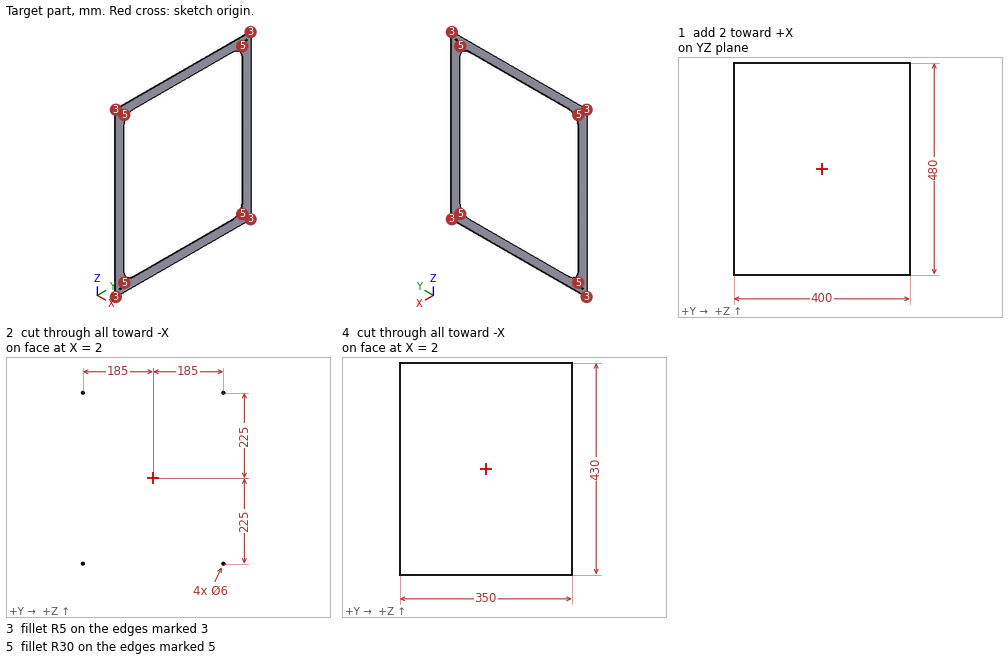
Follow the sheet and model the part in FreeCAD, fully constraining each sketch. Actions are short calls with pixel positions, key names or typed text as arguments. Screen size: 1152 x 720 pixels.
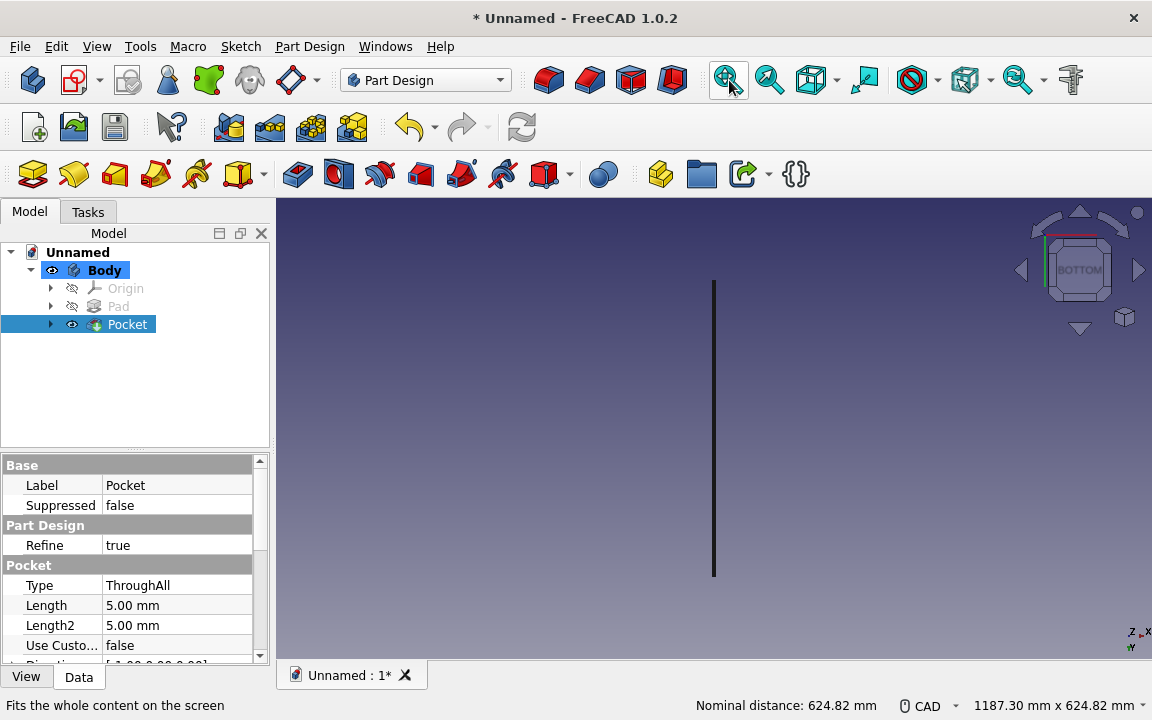
scroll(714, 575, up, 15)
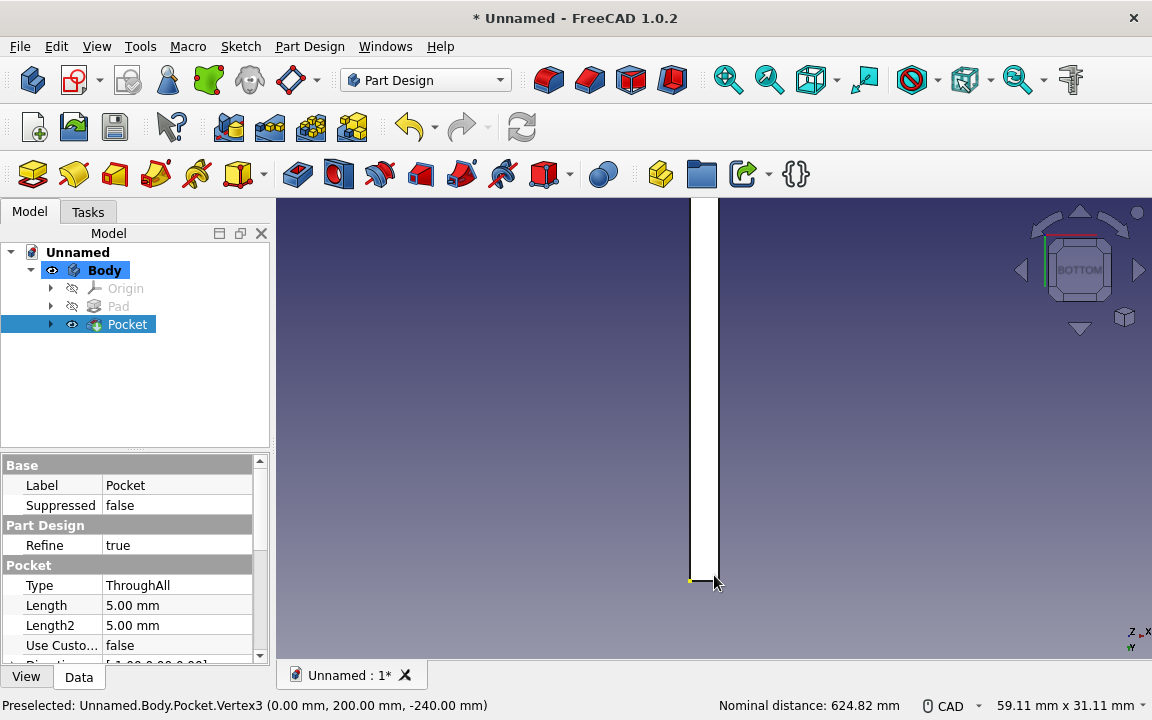
click(704, 580, ctrl)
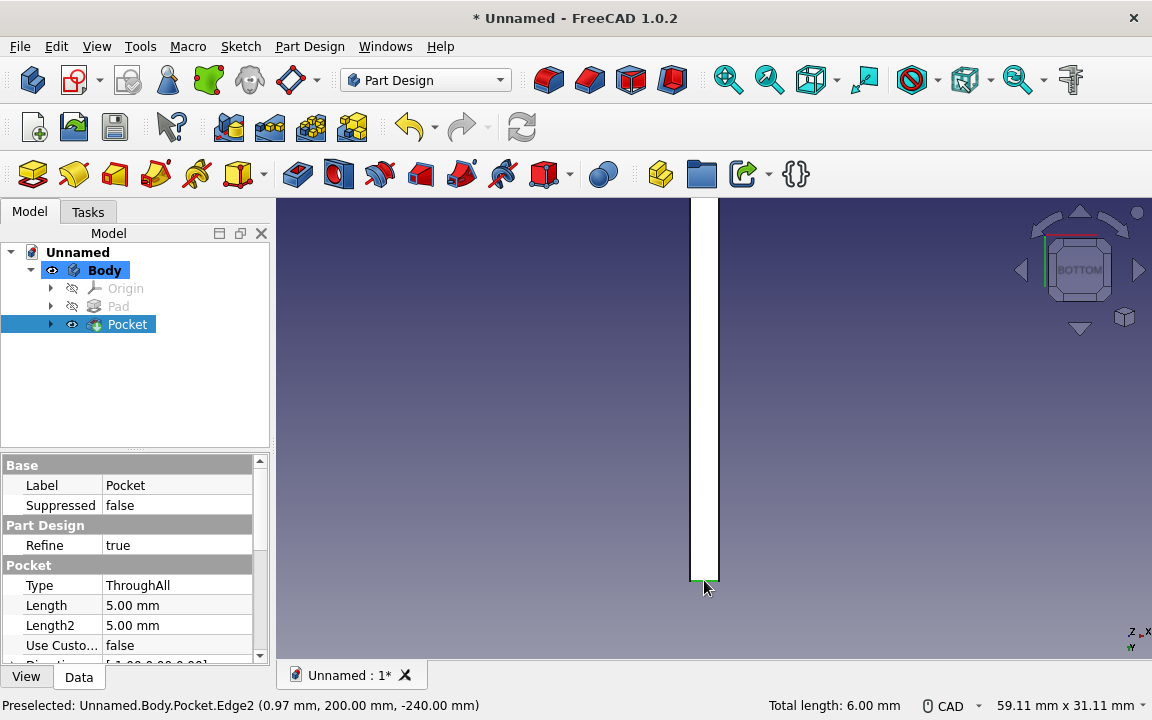
click(729, 80)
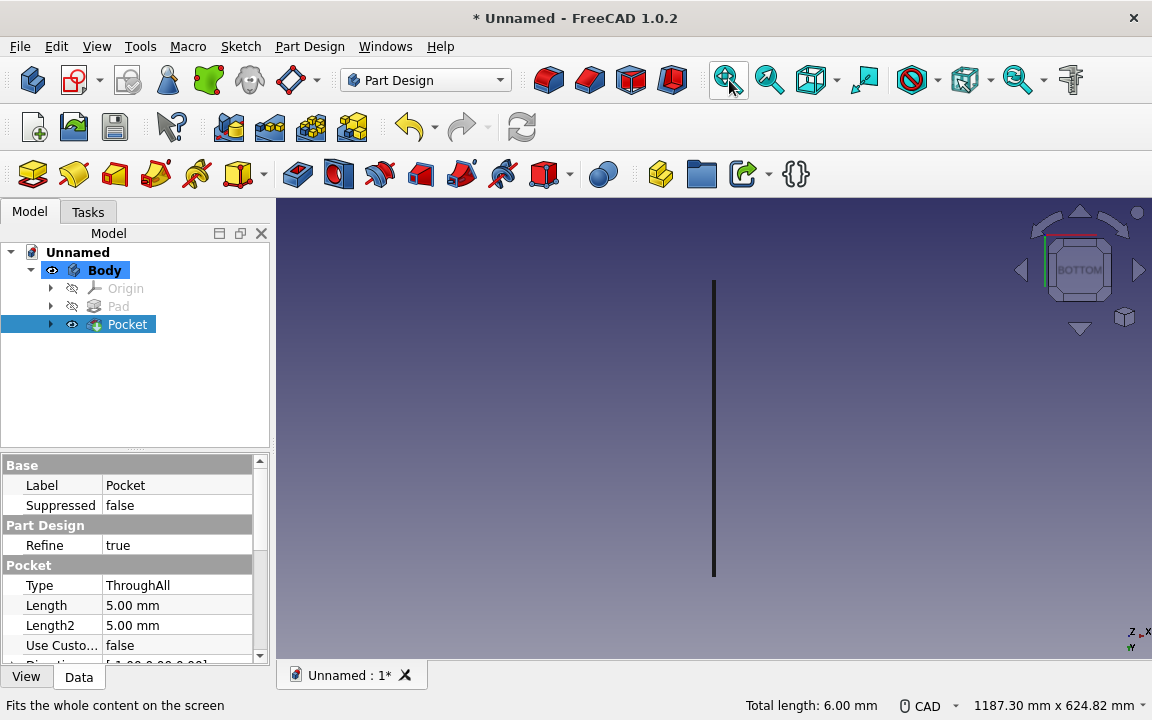
key(4)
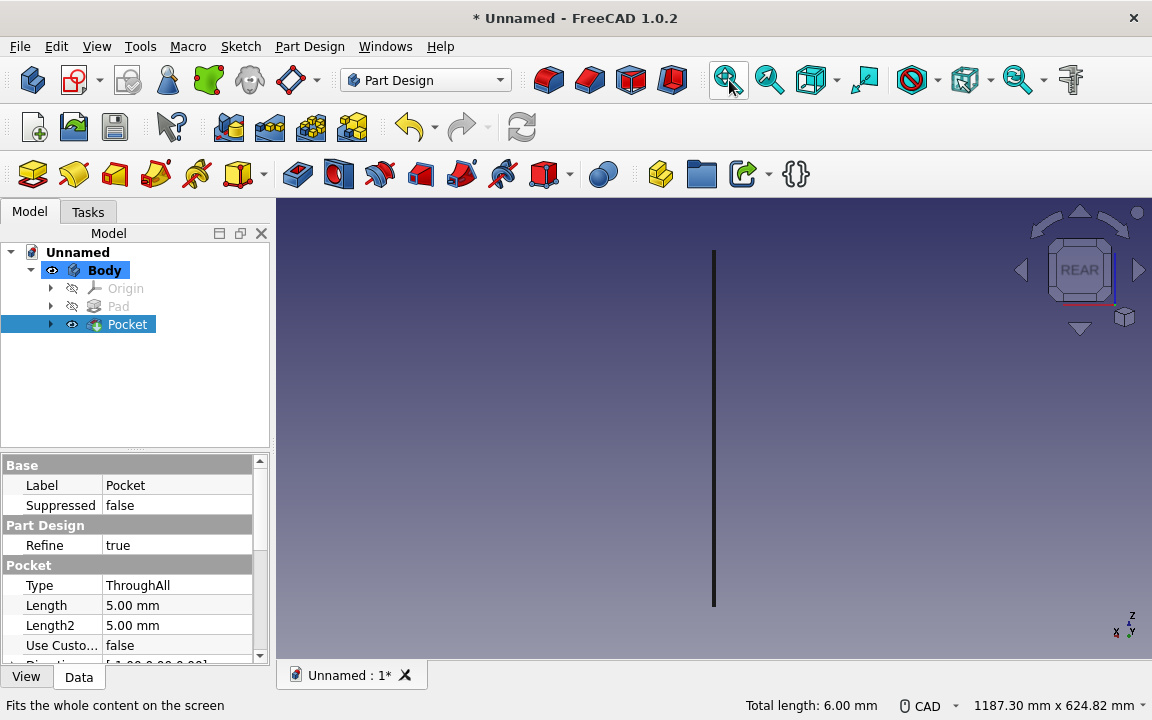
scroll(714, 250, up, 15)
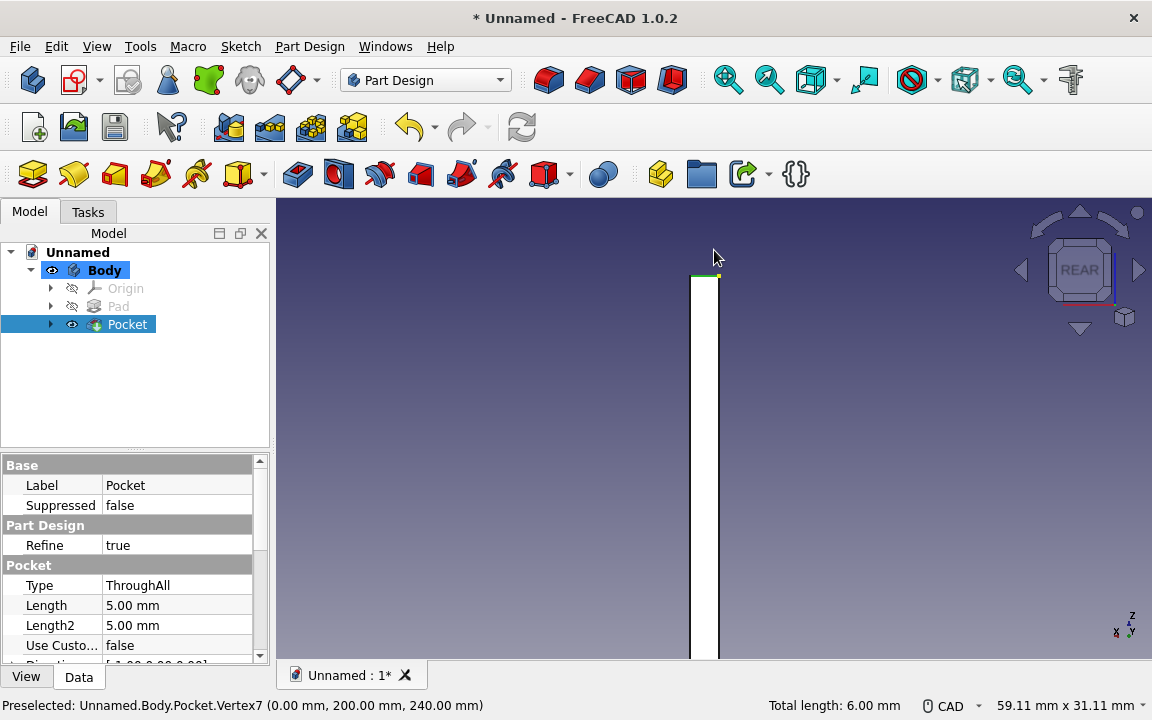
click(729, 80)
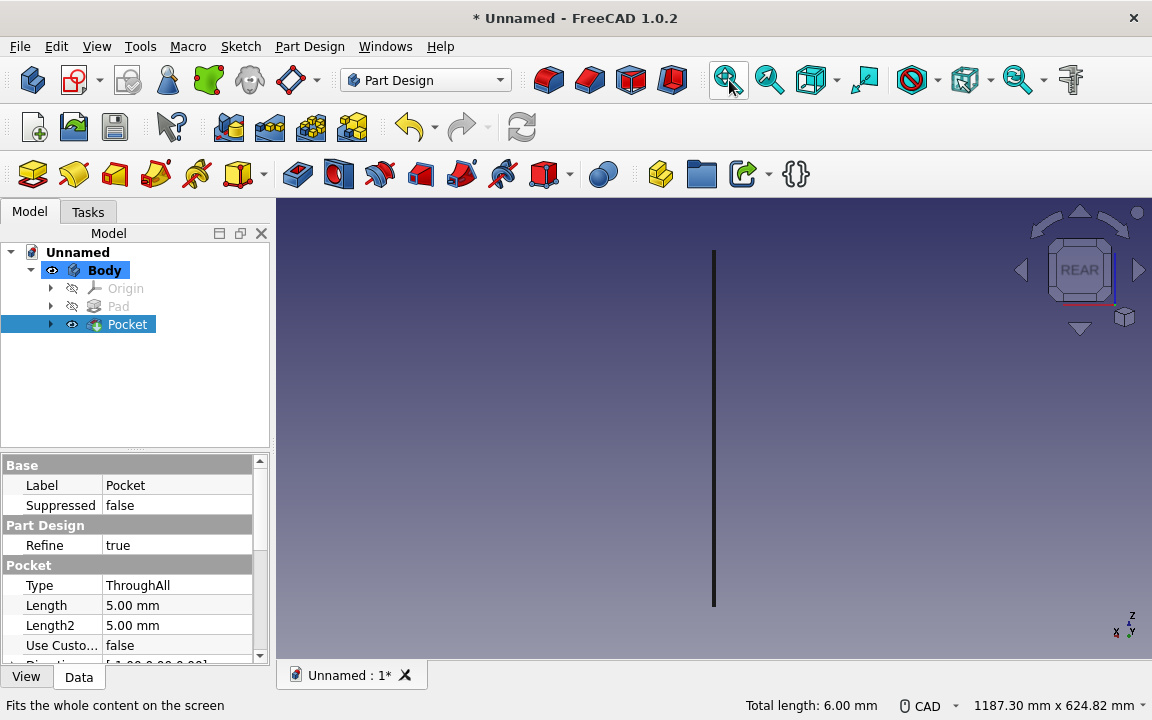
key(6)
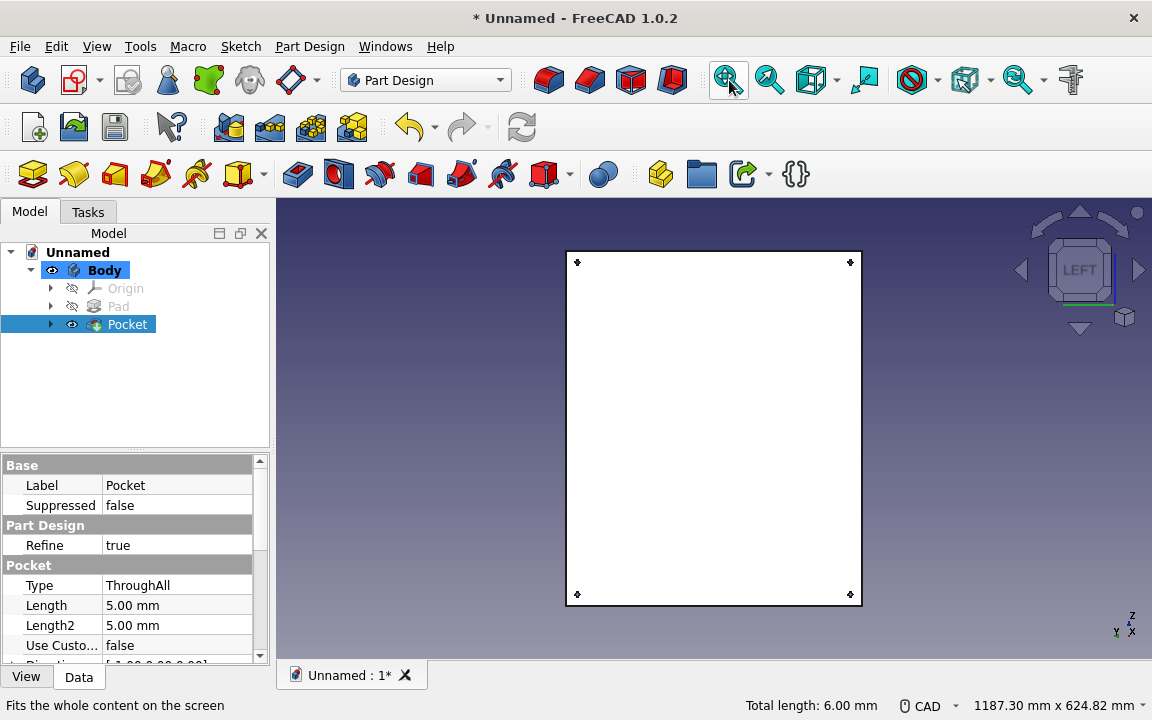
scroll(862, 250, up, 15)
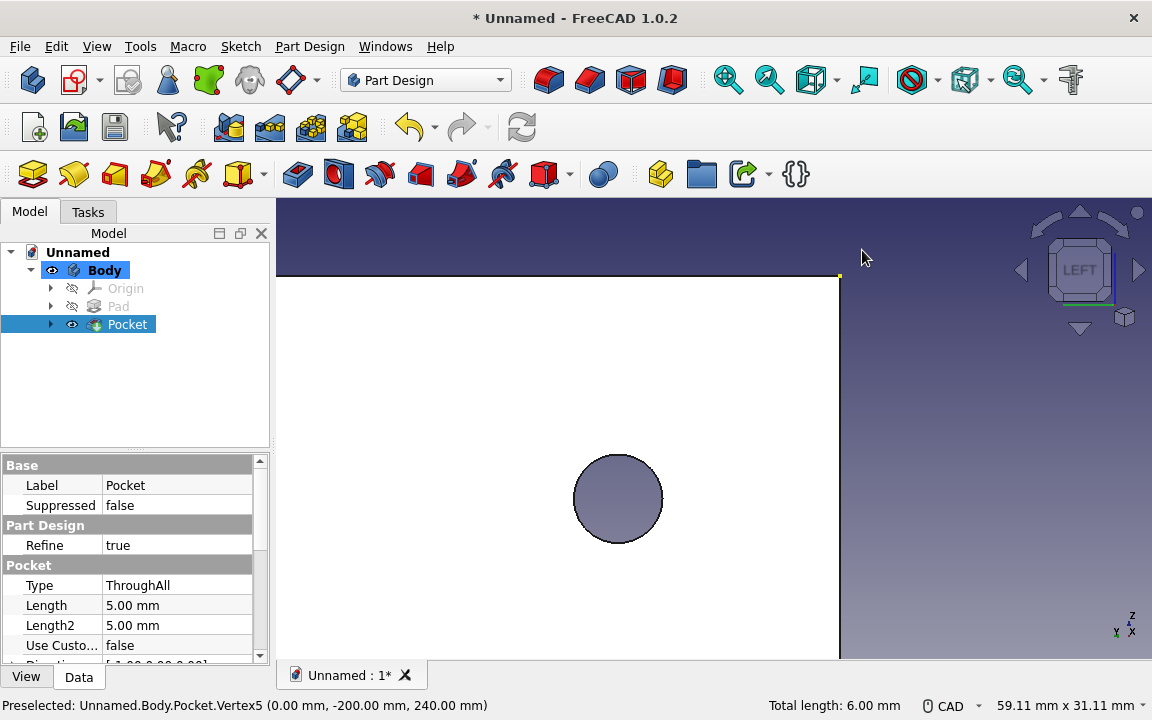
click(729, 80)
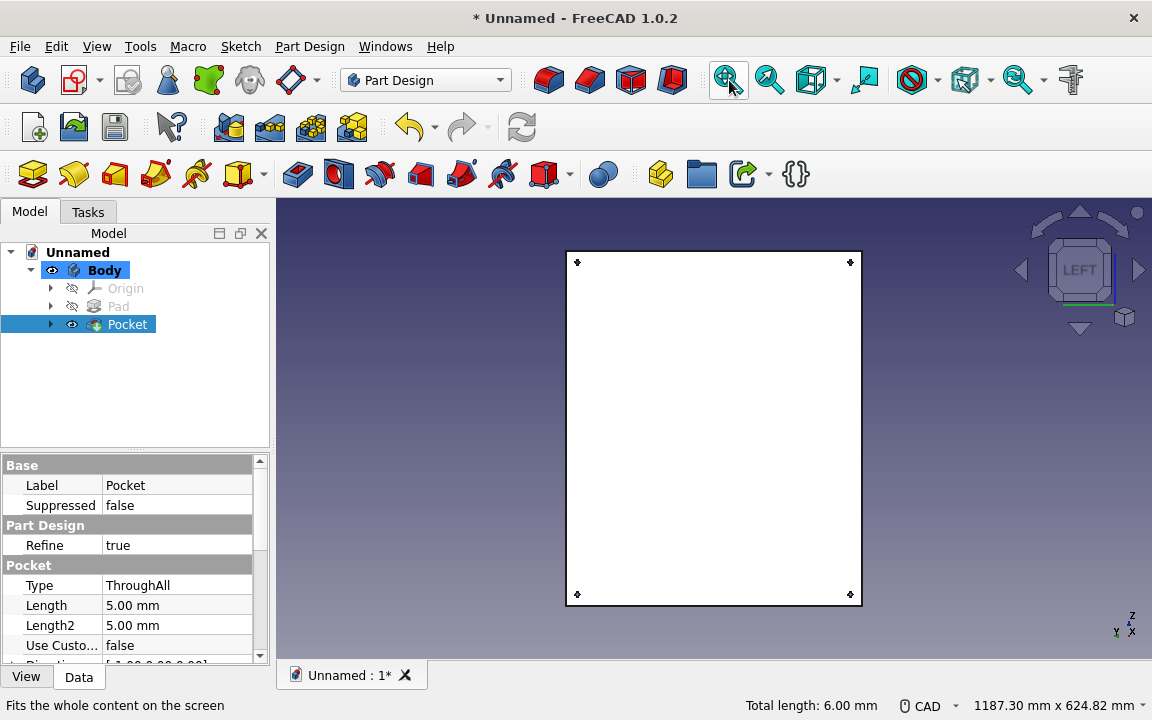
key(v)
key(3)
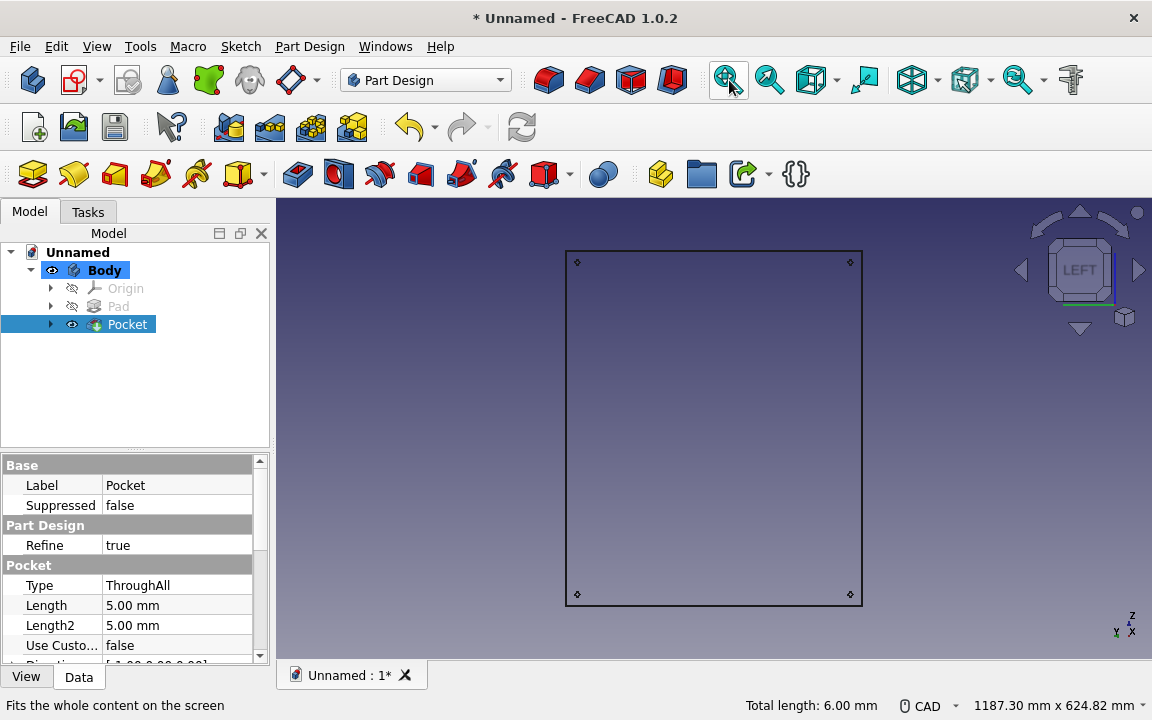
key(0)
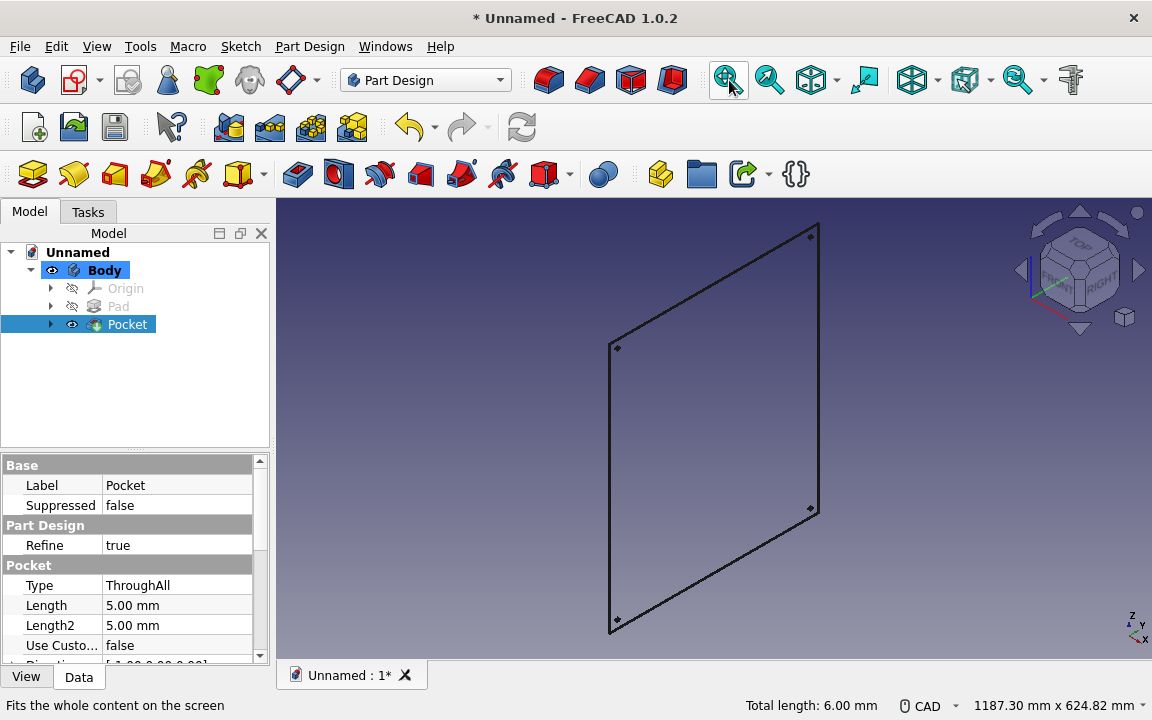
scroll(610, 343, up, 15)